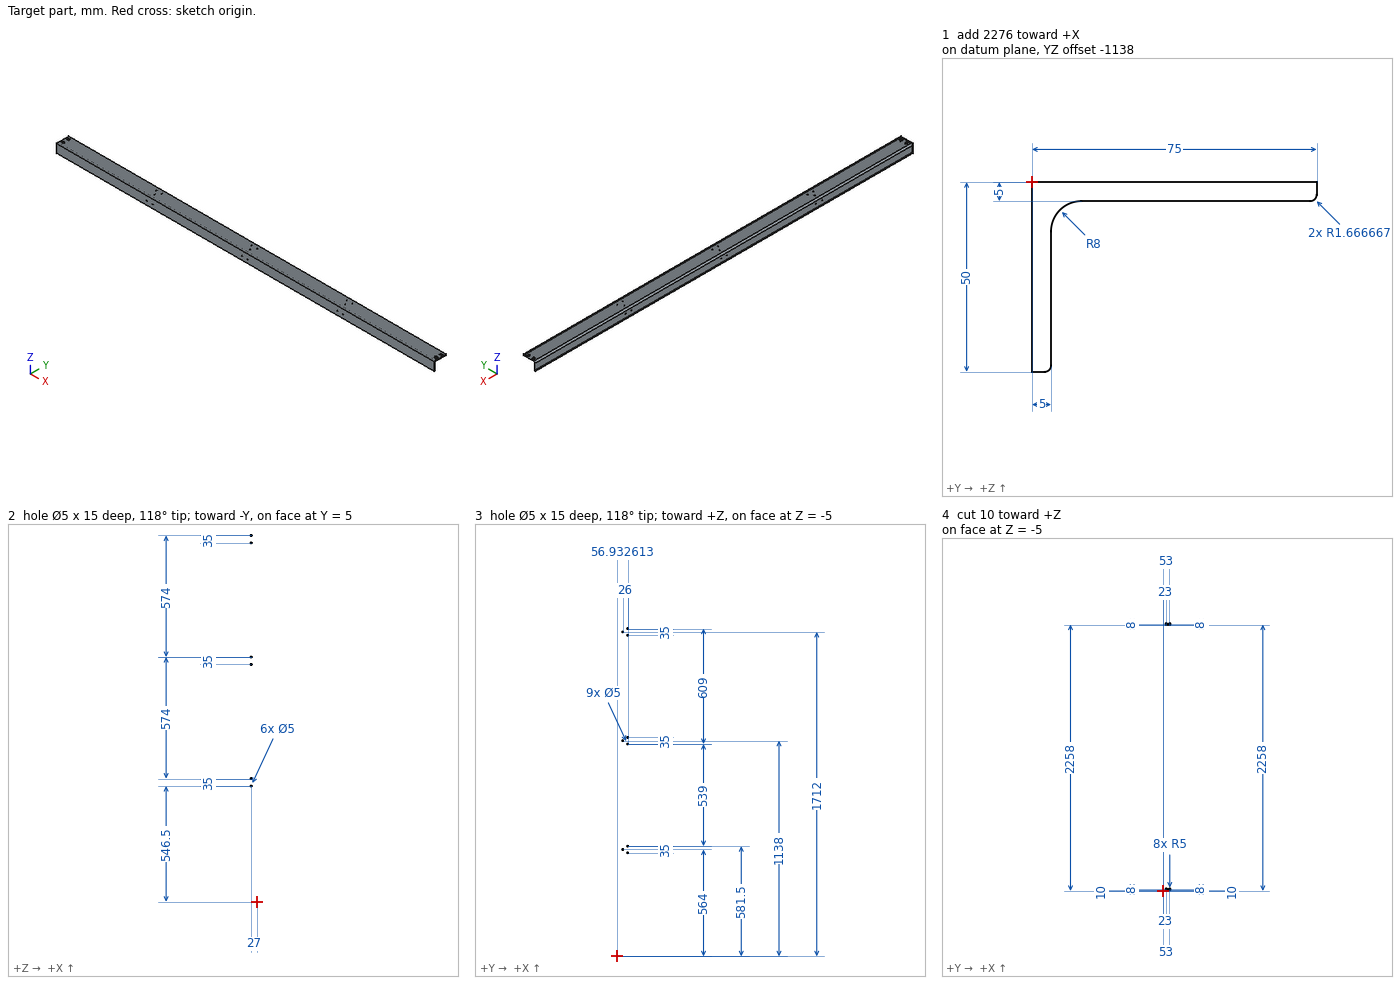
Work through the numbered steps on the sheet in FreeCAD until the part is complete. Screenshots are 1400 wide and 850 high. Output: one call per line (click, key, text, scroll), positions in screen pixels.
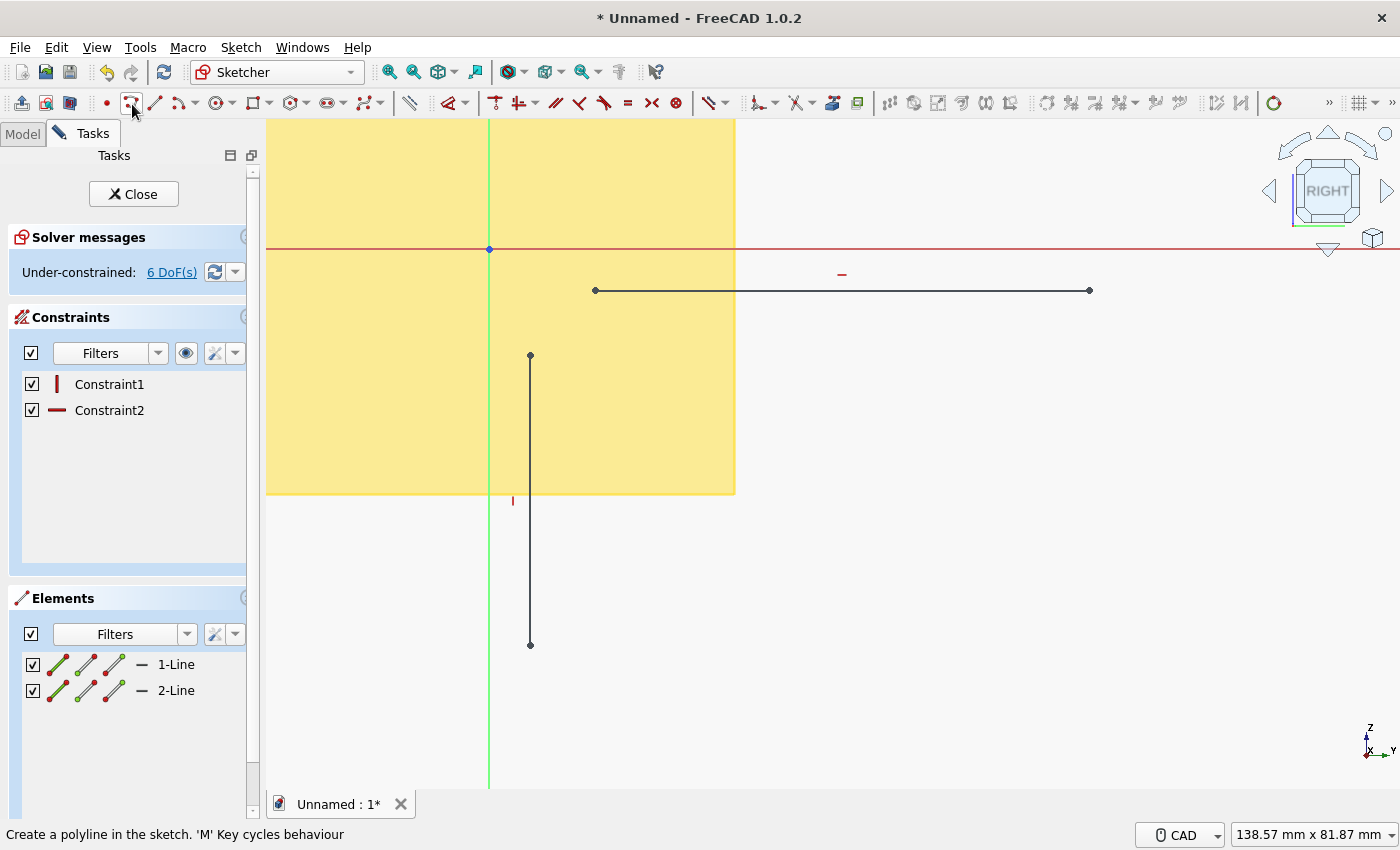
click(1103, 276)
click(1103, 249)
click(489, 249)
click(498, 658)
click(516, 658)
right_click(516, 658)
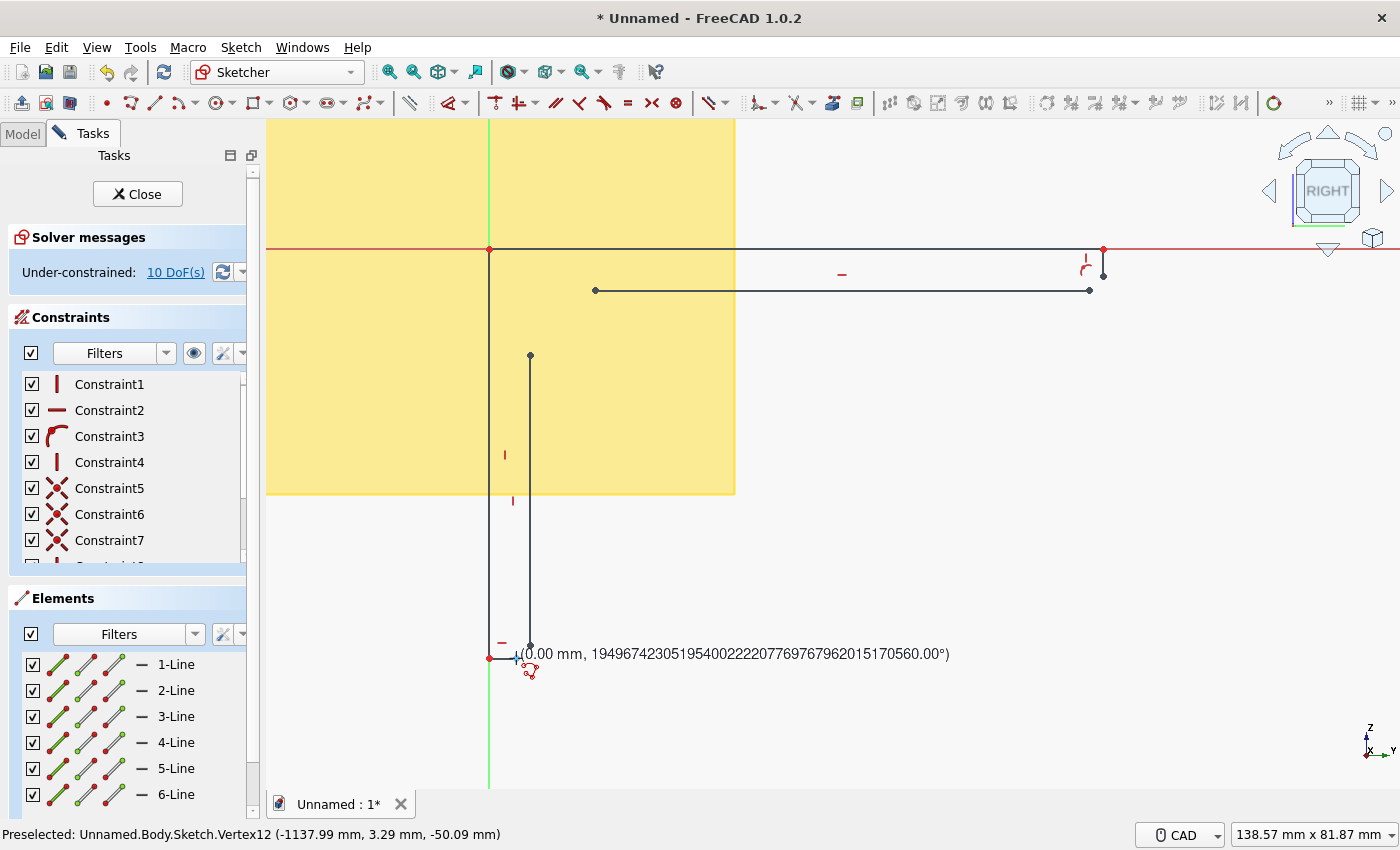
key(g)
key(3)
key(a)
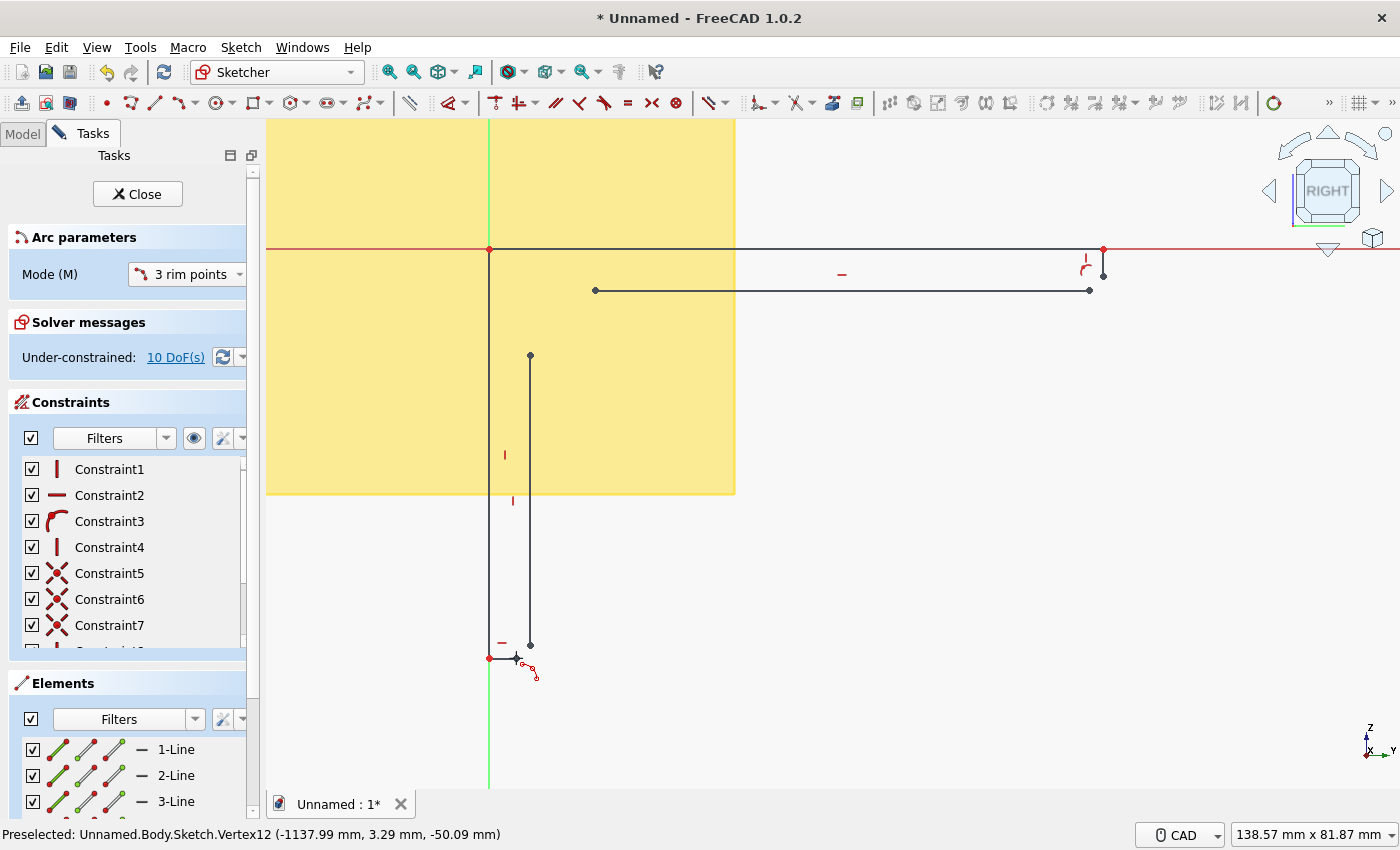
click(530, 356)
click(595, 291)
click(549, 309)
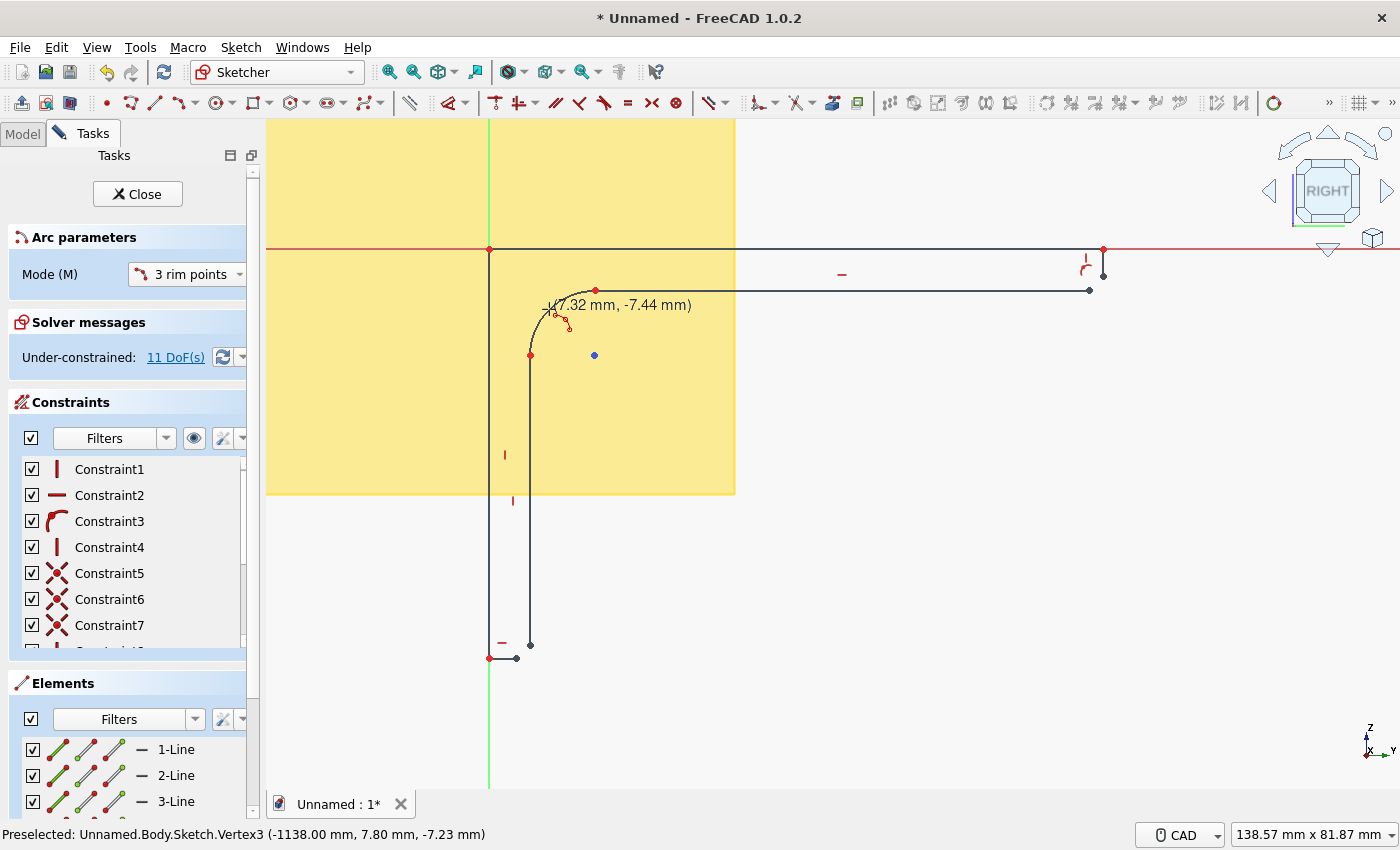
click(1089, 291)
click(1103, 277)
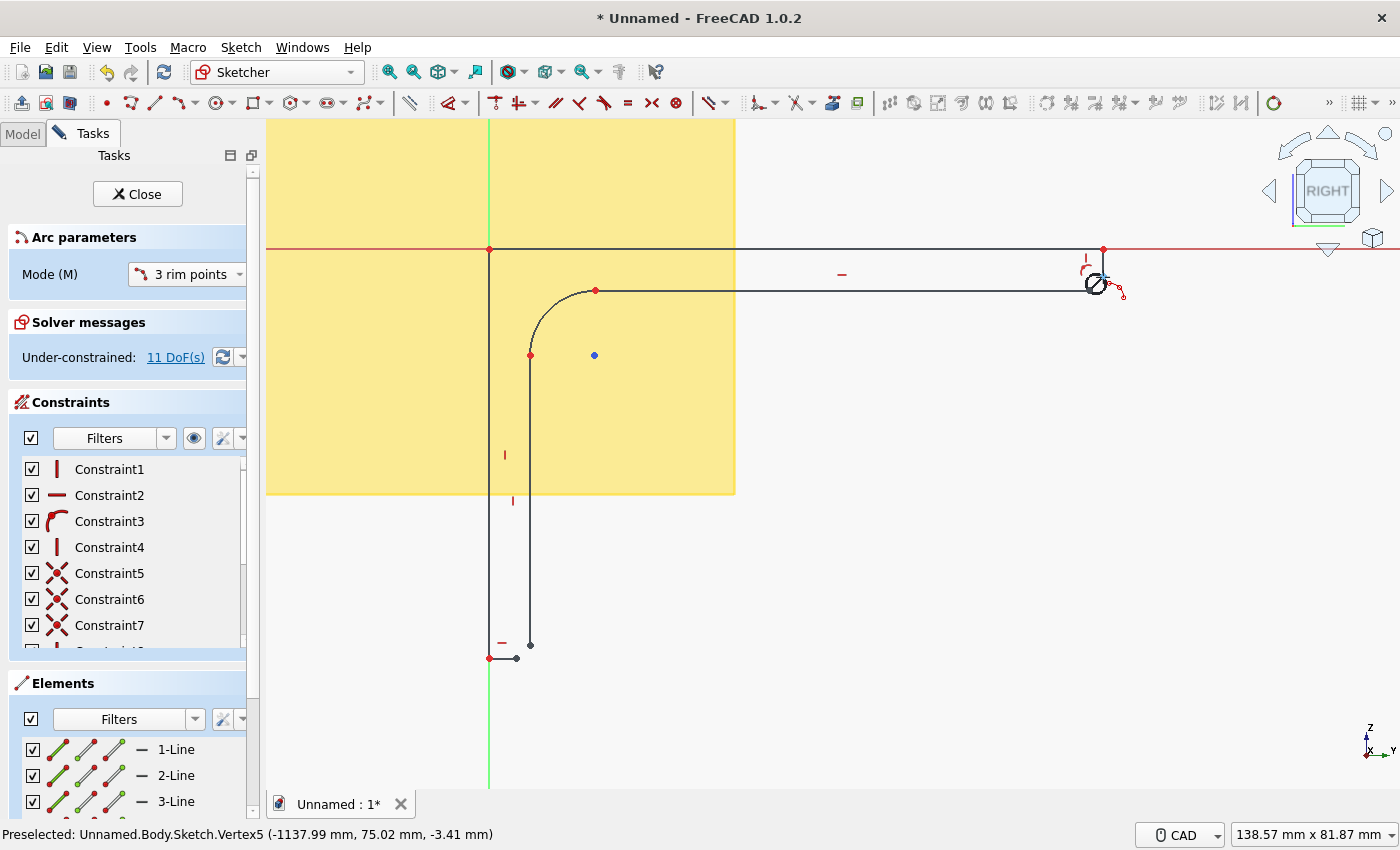
scroll(1099, 286, up, 7)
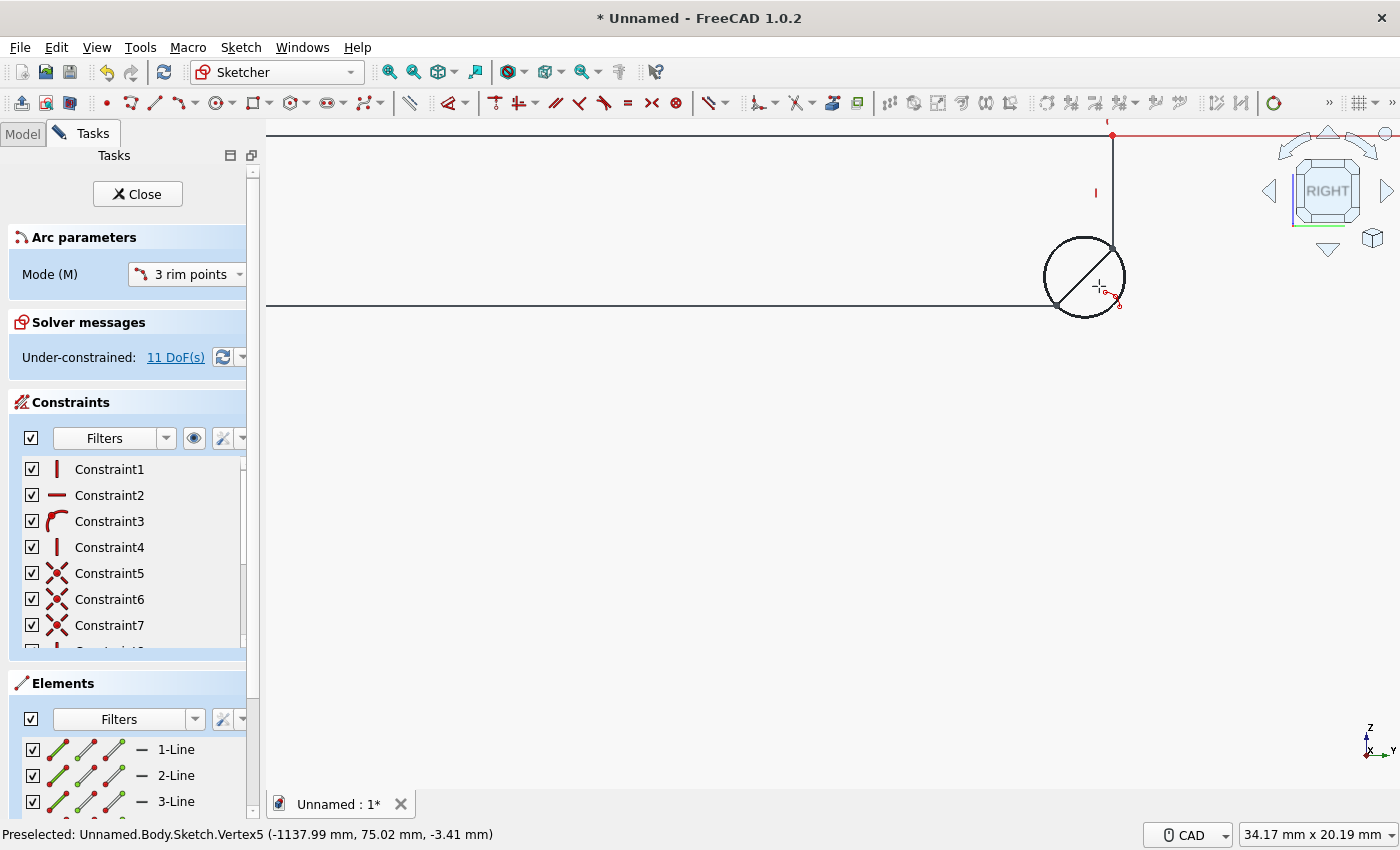
click(1096, 285)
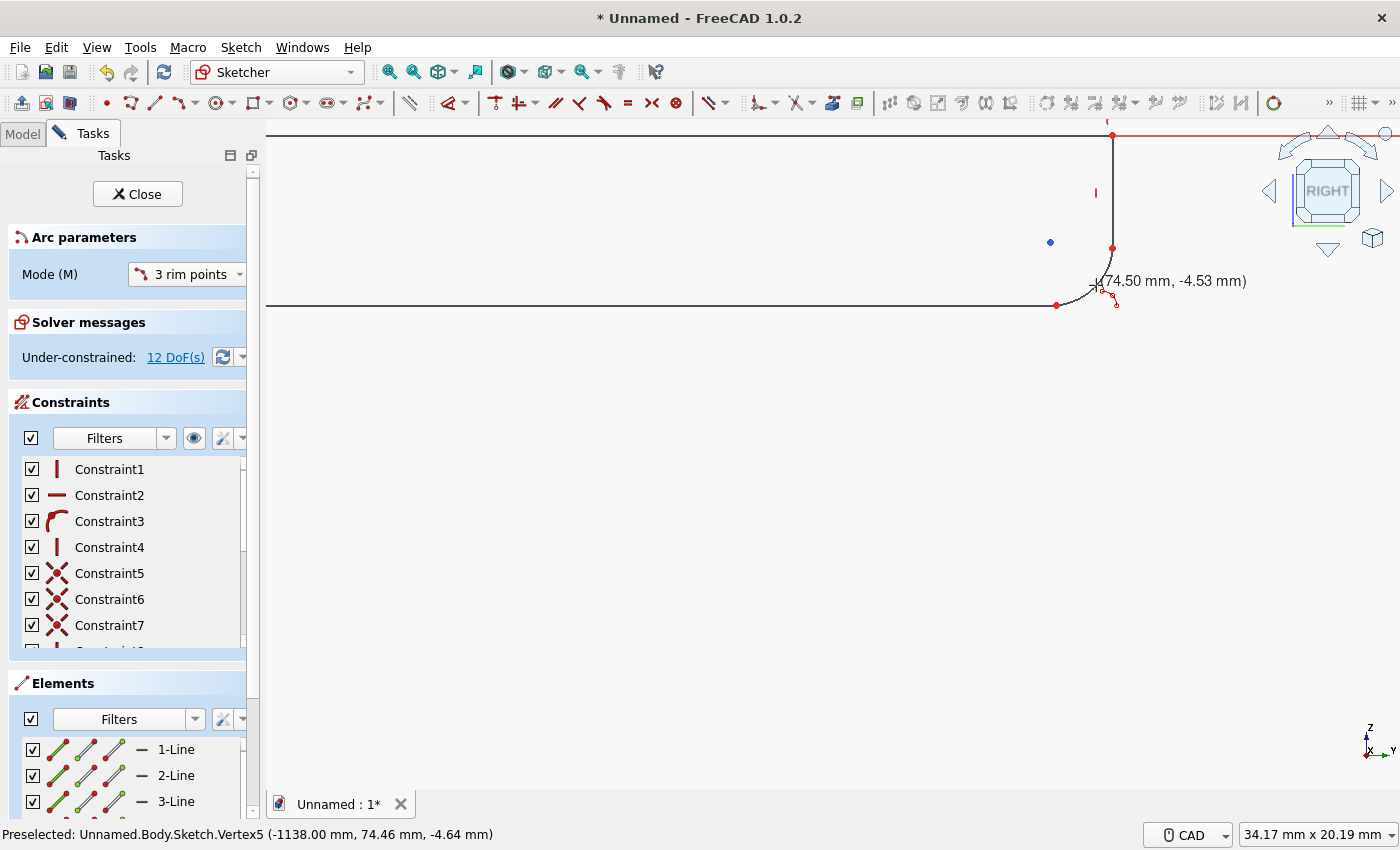
scroll(1058, 287, down, 7)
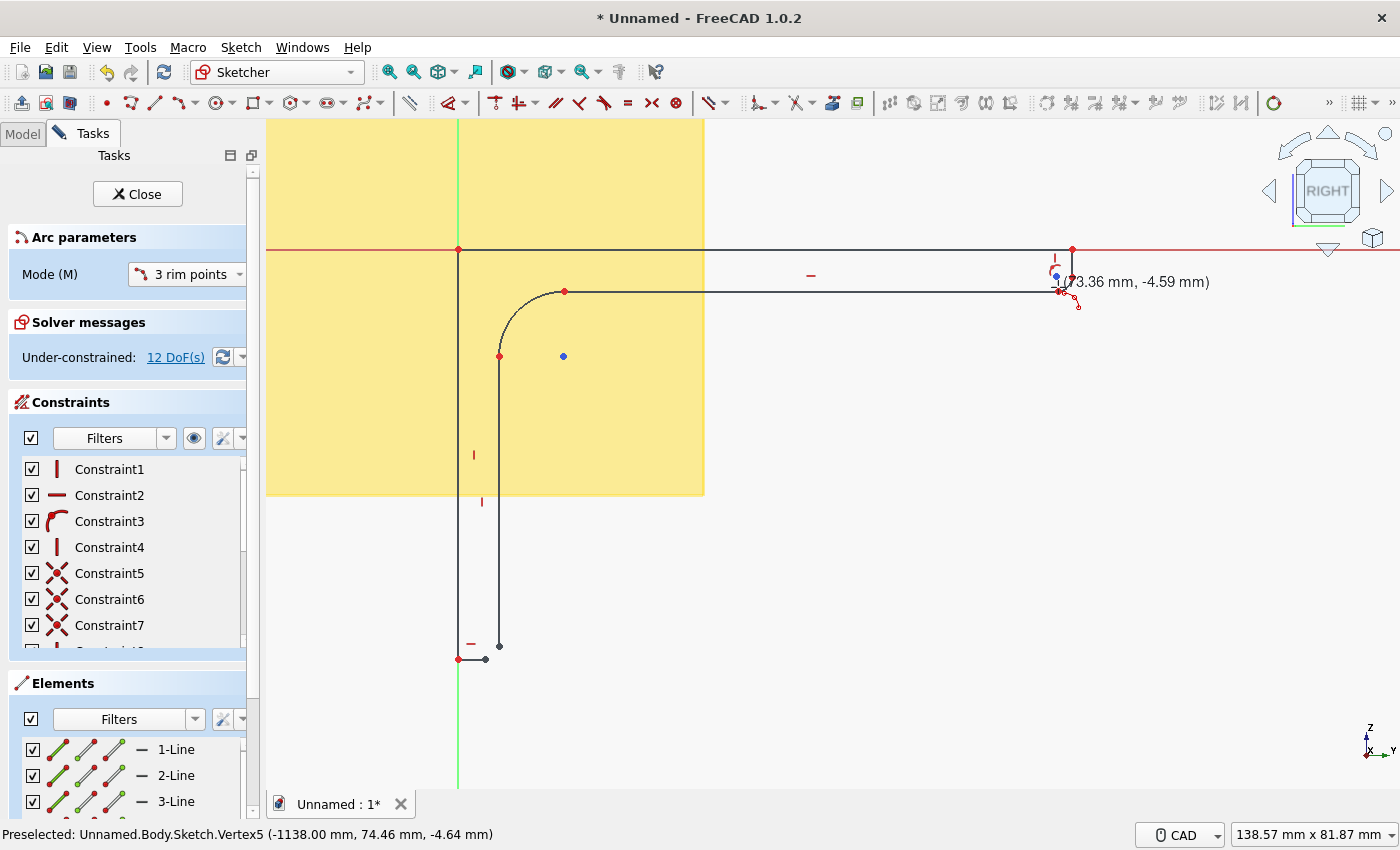
click(485, 660)
click(499, 647)